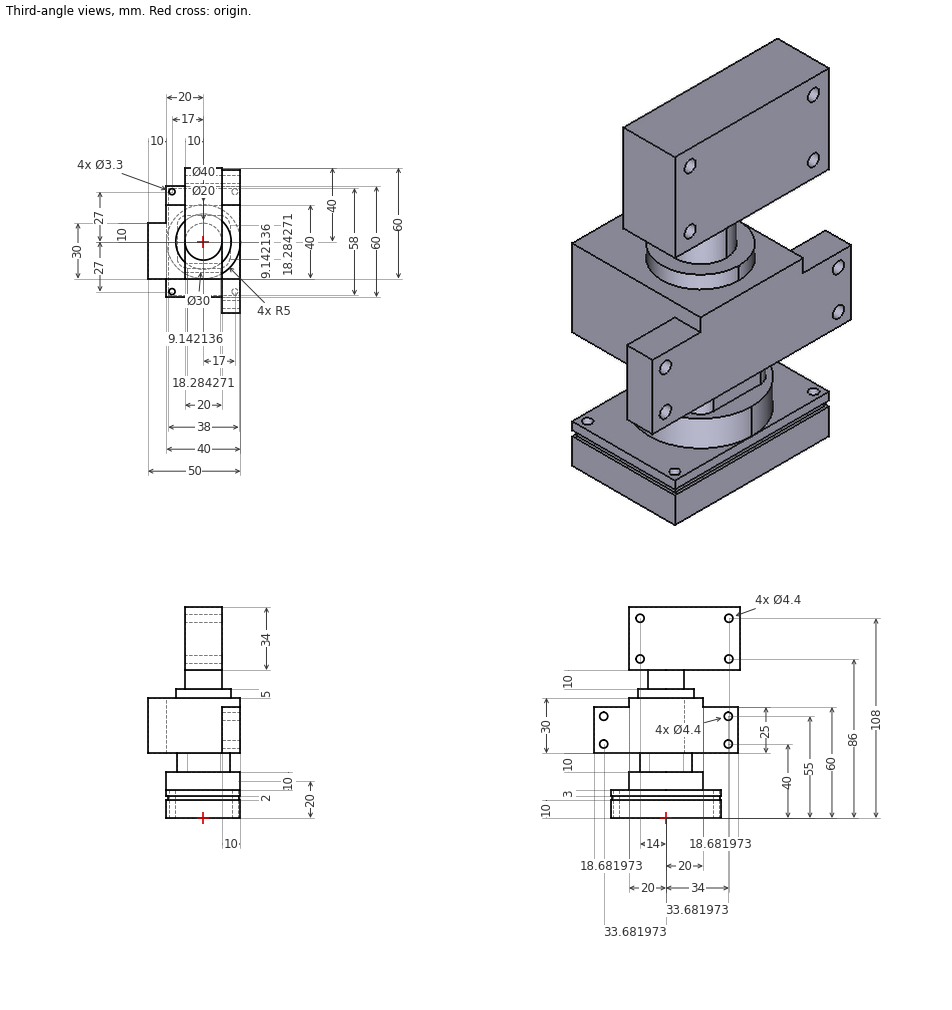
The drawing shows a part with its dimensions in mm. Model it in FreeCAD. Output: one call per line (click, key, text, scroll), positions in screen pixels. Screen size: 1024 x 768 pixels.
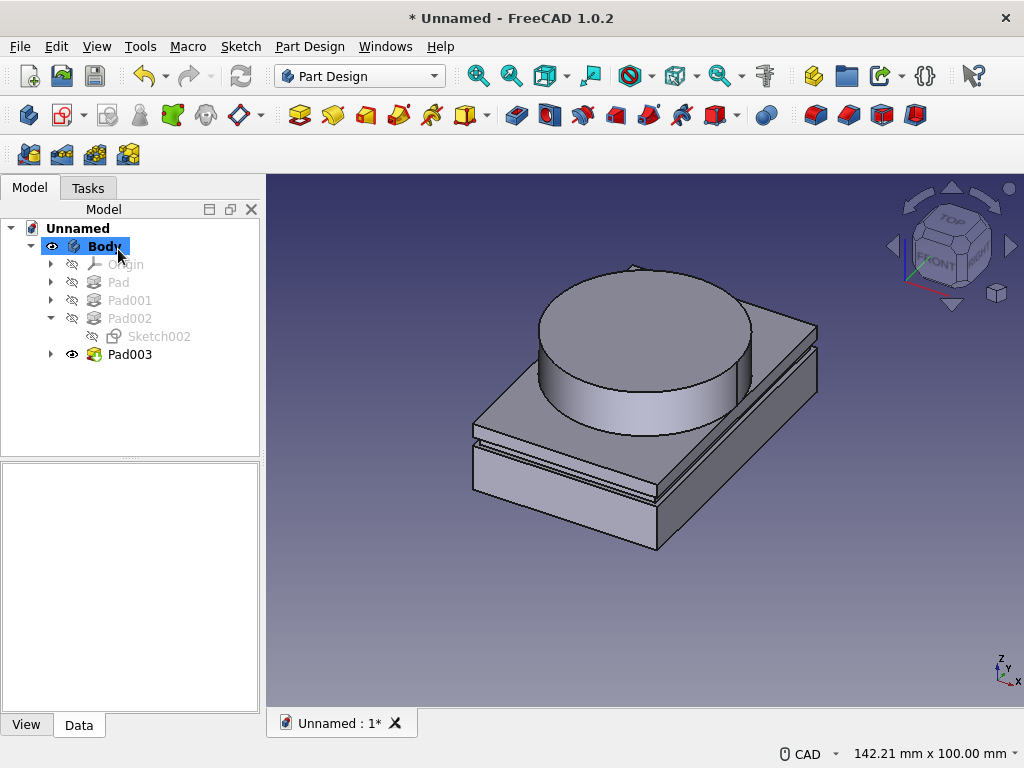
click(645, 330)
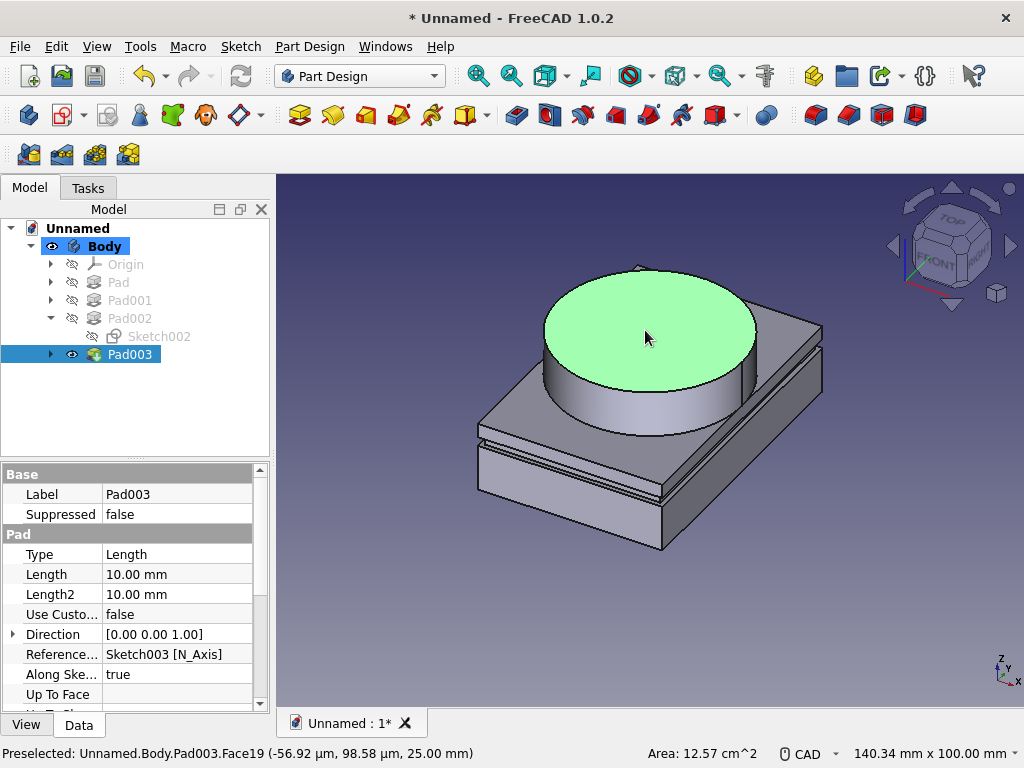
click(62, 116)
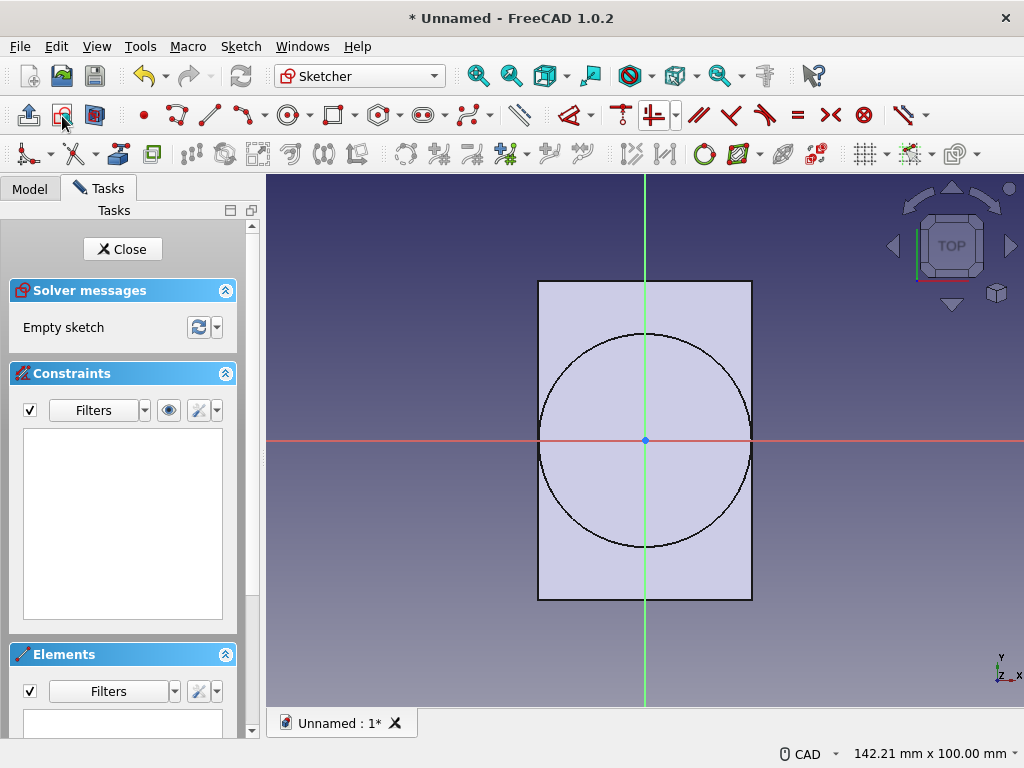
scroll(701, 440, up, 4)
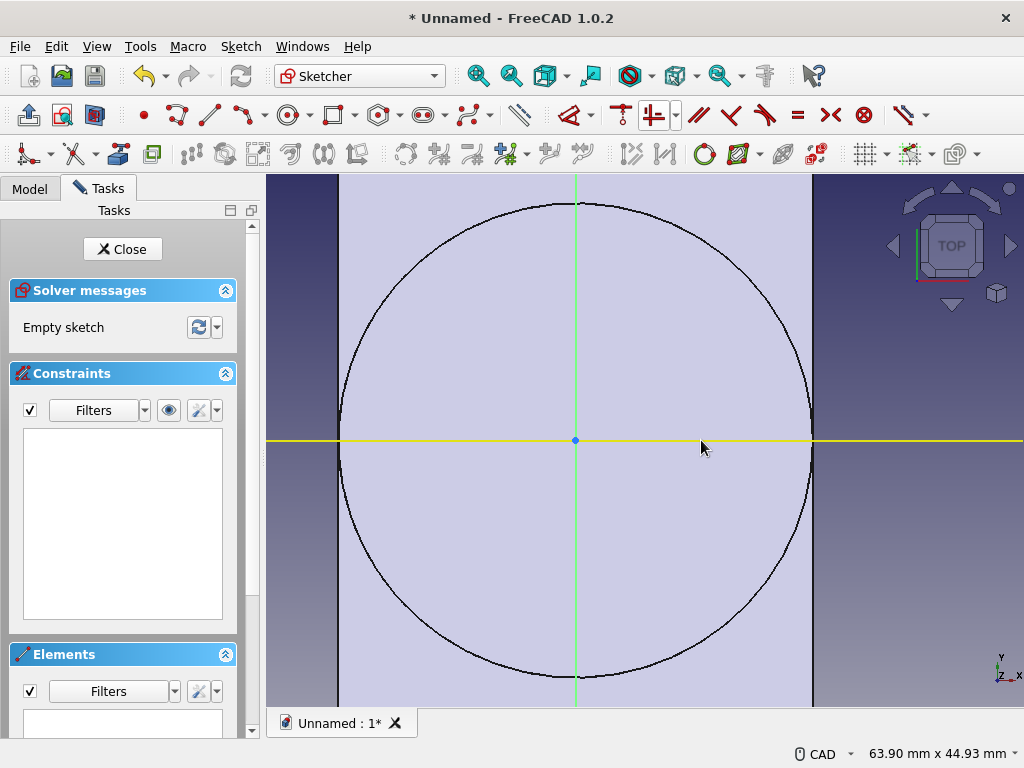
click(210, 116)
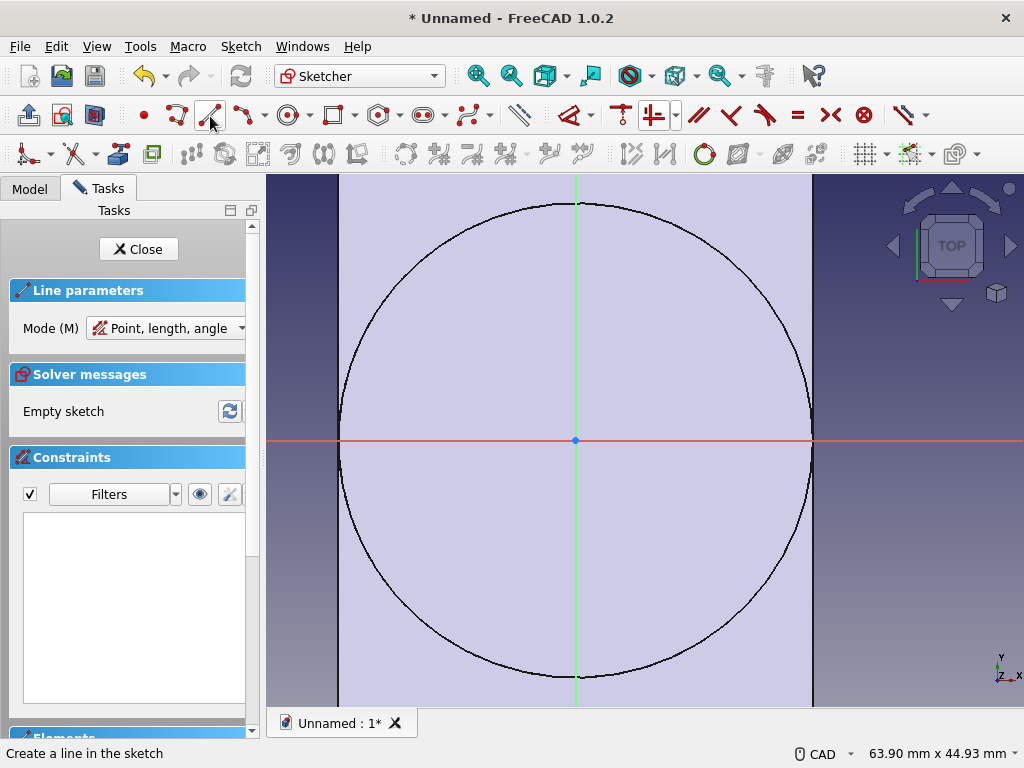
click(467, 608)
click(684, 608)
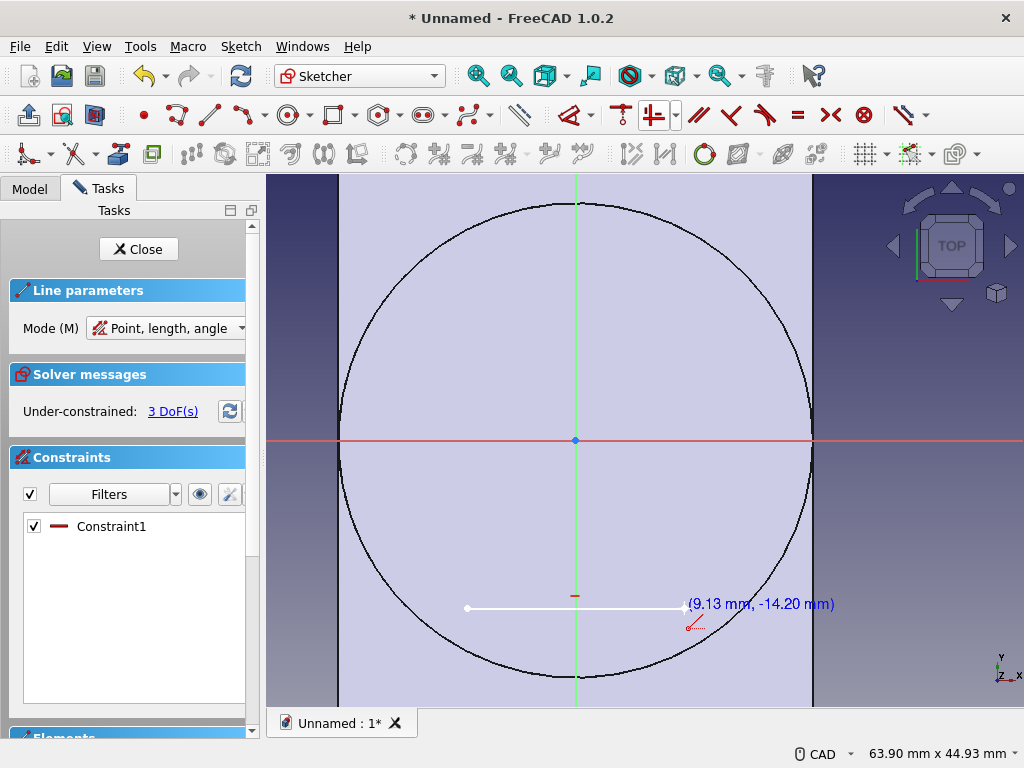
click(743, 549)
click(743, 332)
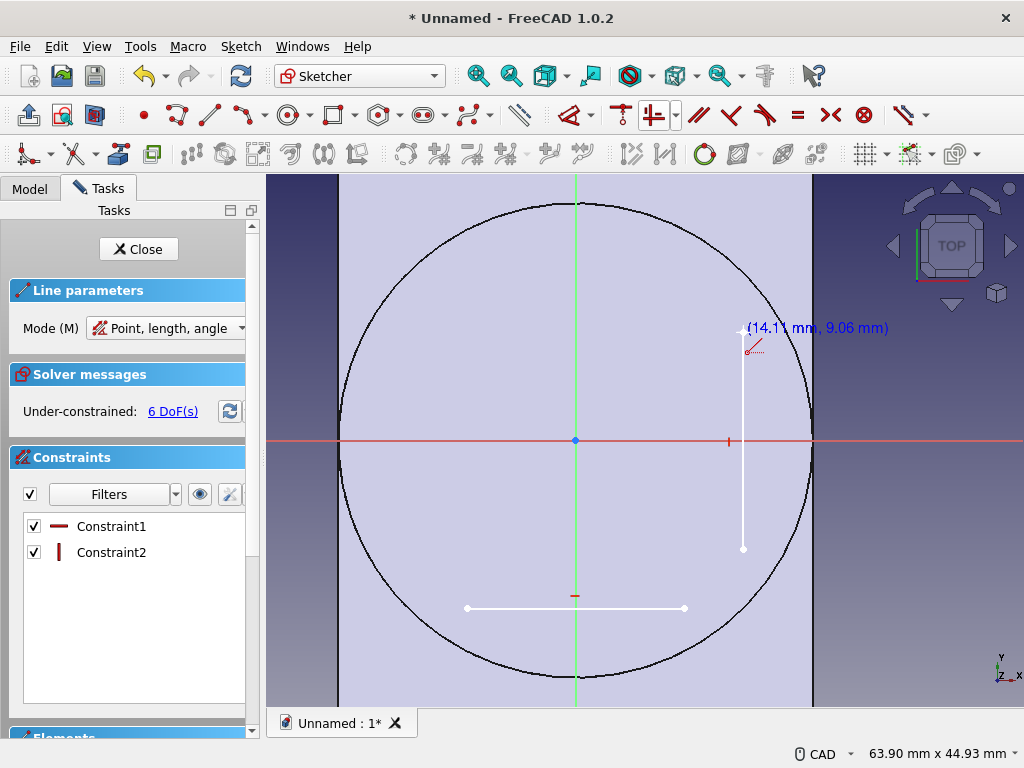
click(684, 273)
click(467, 273)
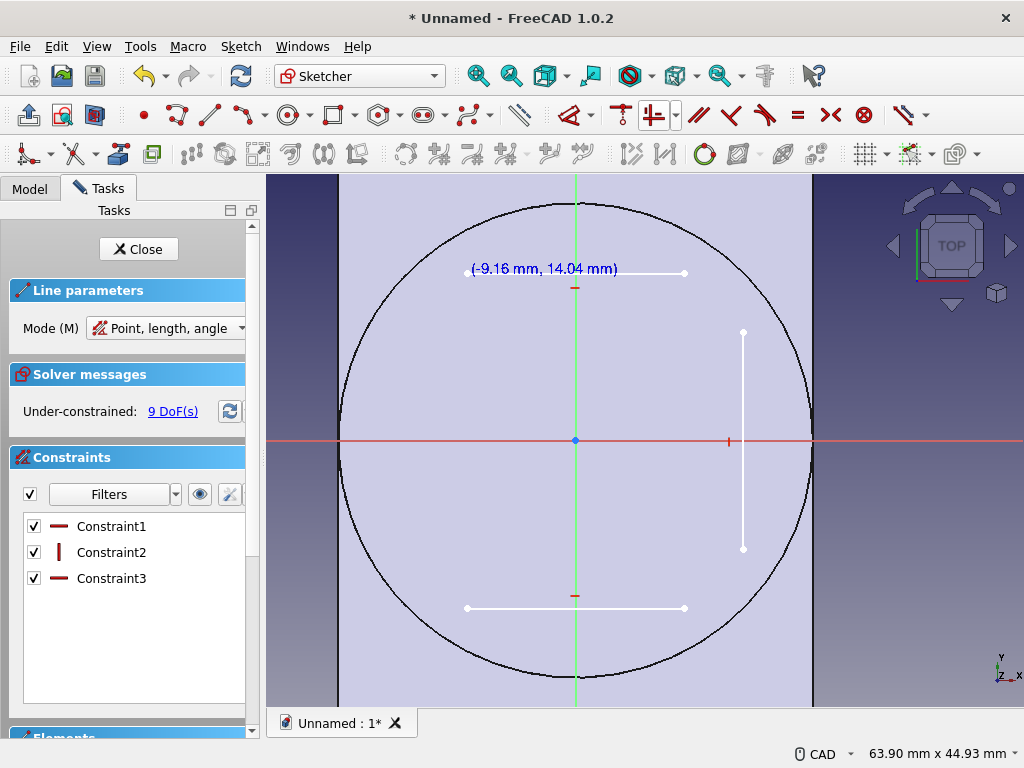
click(408, 332)
click(408, 549)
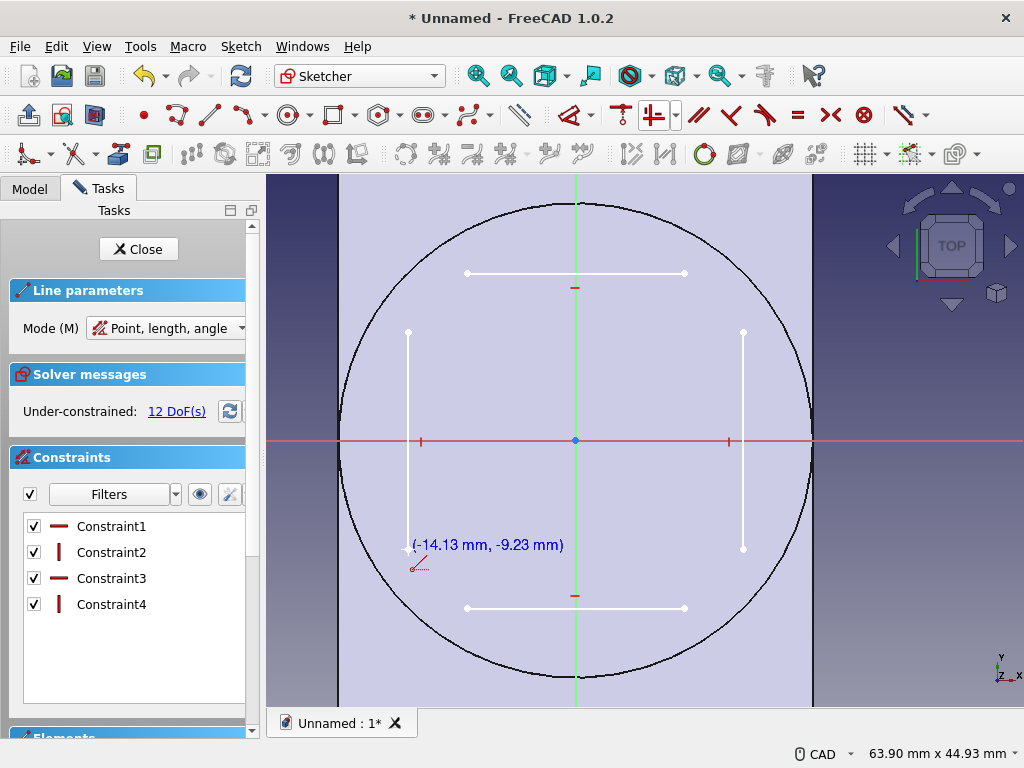
click(242, 116)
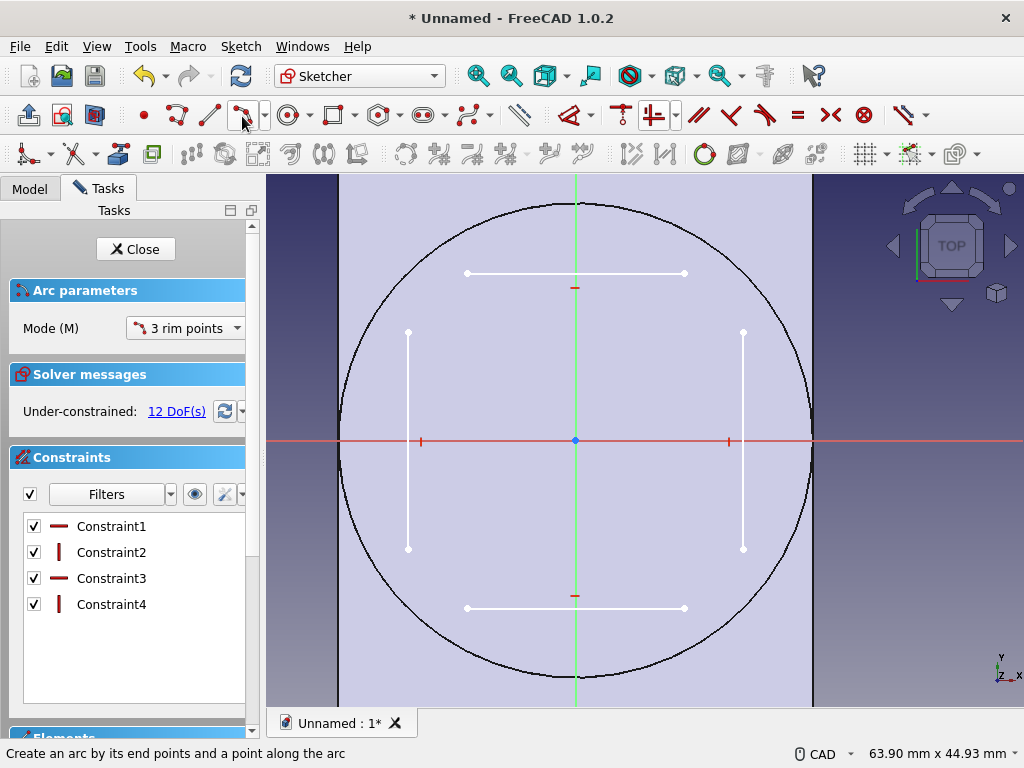
click(684, 609)
click(743, 550)
click(726, 591)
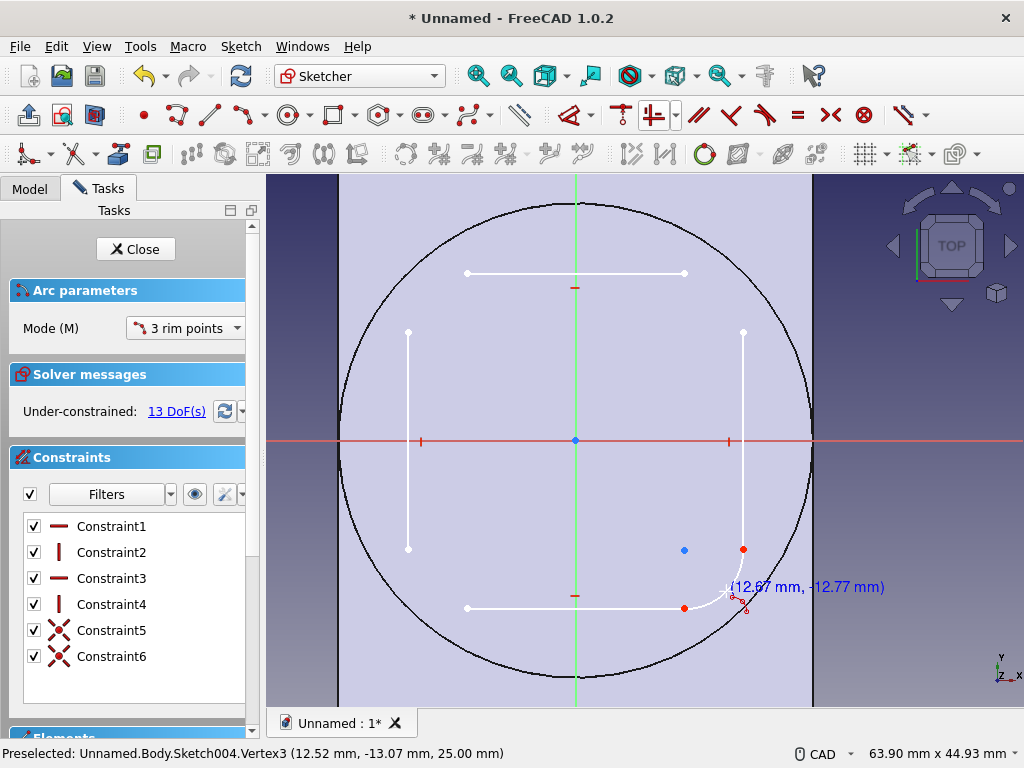
click(743, 333)
click(684, 274)
click(726, 290)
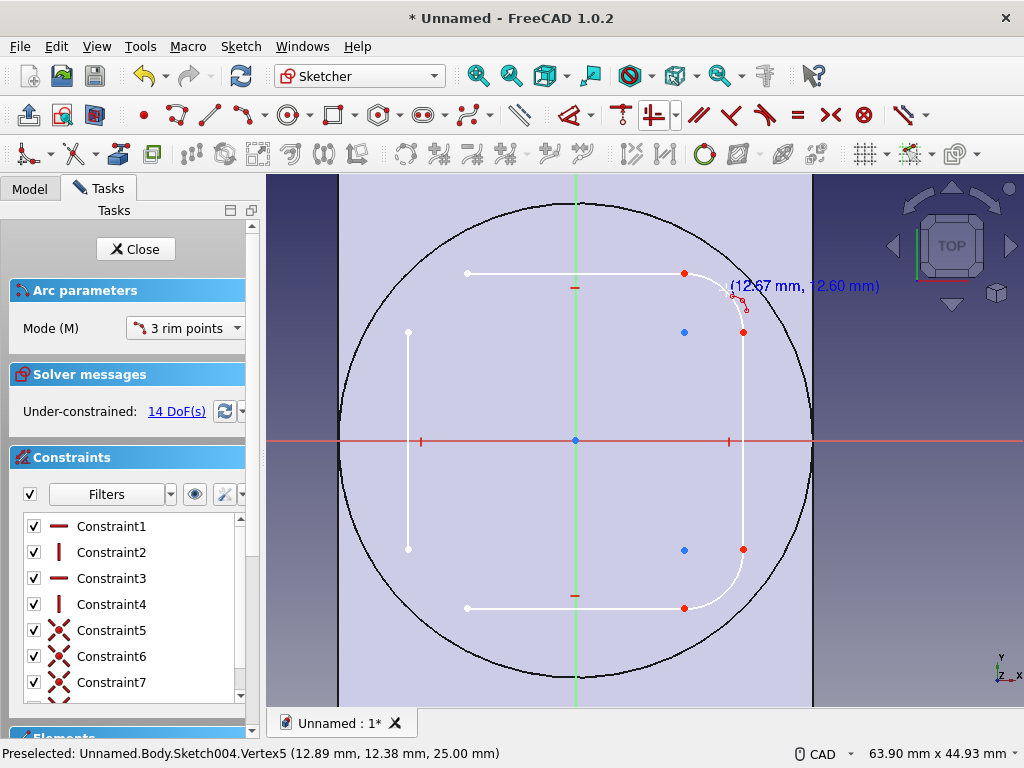
click(467, 274)
click(408, 333)
click(425, 290)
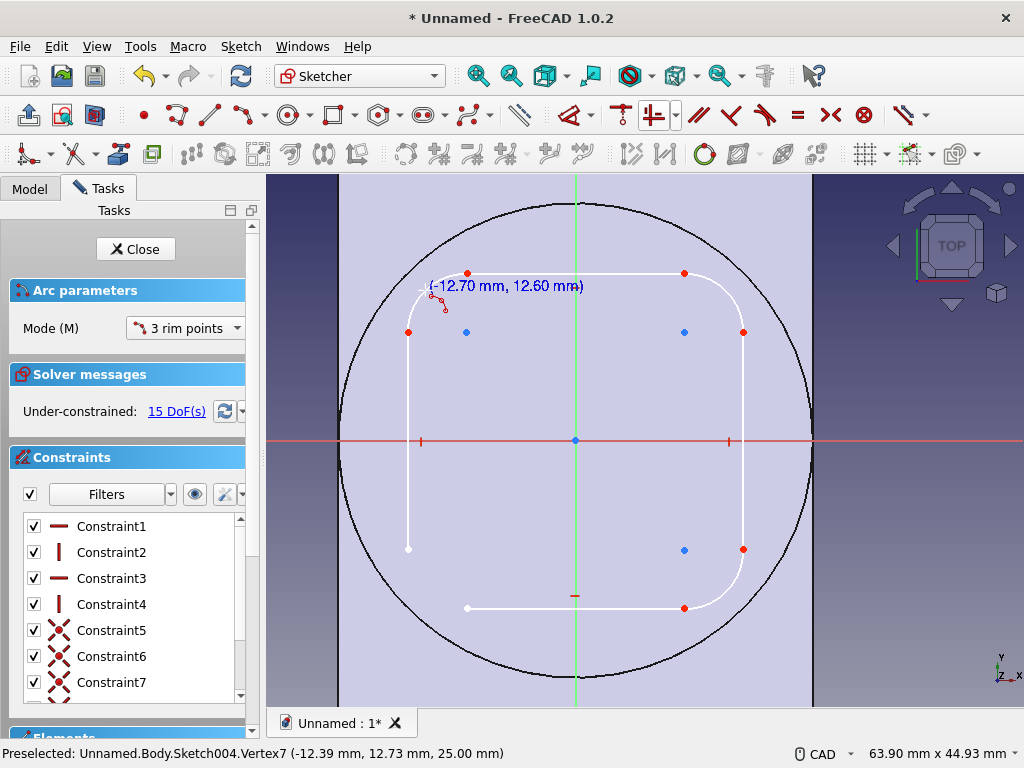
click(408, 550)
click(467, 609)
click(425, 591)
key(Escape)